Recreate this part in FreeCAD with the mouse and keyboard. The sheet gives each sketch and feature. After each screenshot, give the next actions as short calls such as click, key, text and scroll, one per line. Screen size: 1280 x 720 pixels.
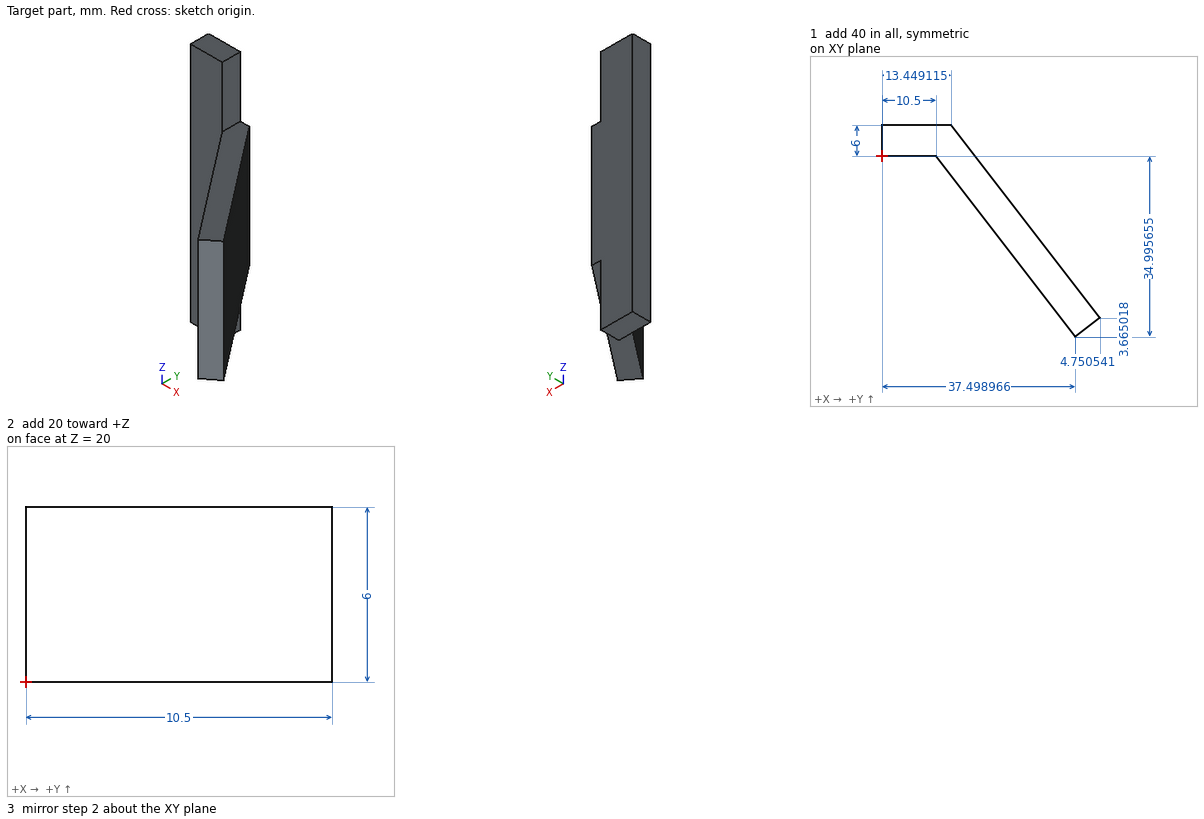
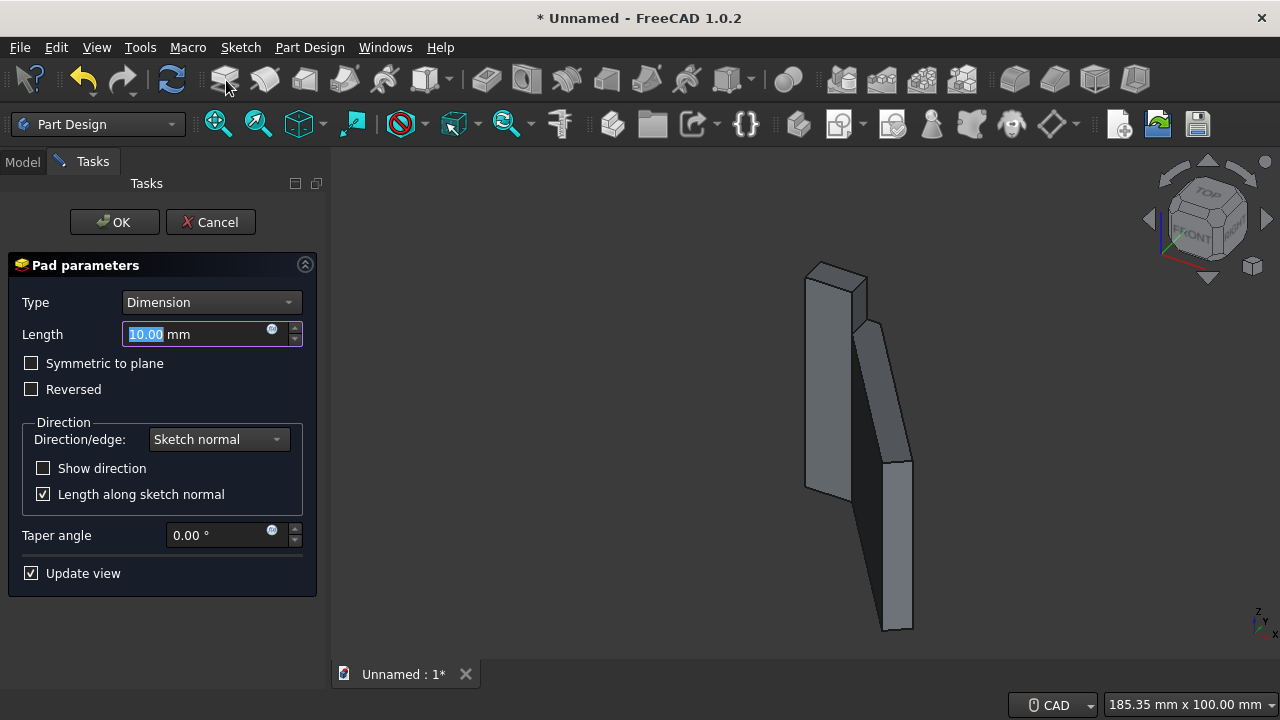
text(20)
key(Tab)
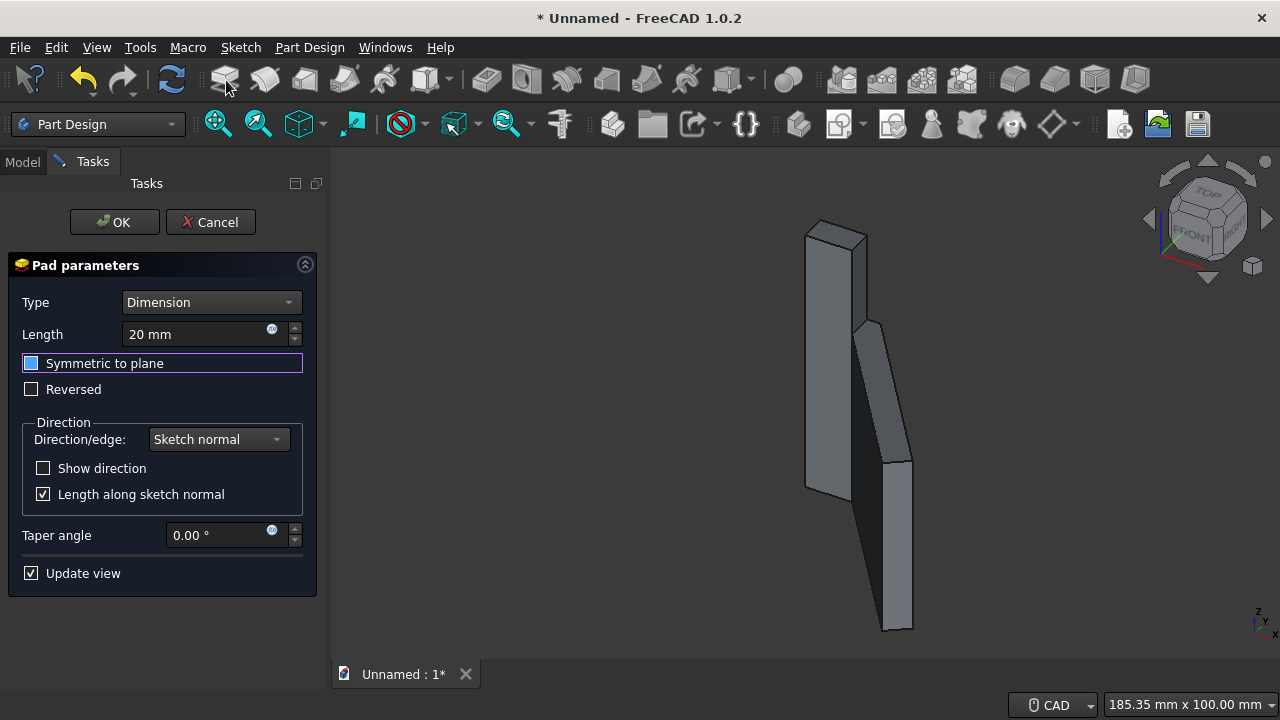
click(115, 222)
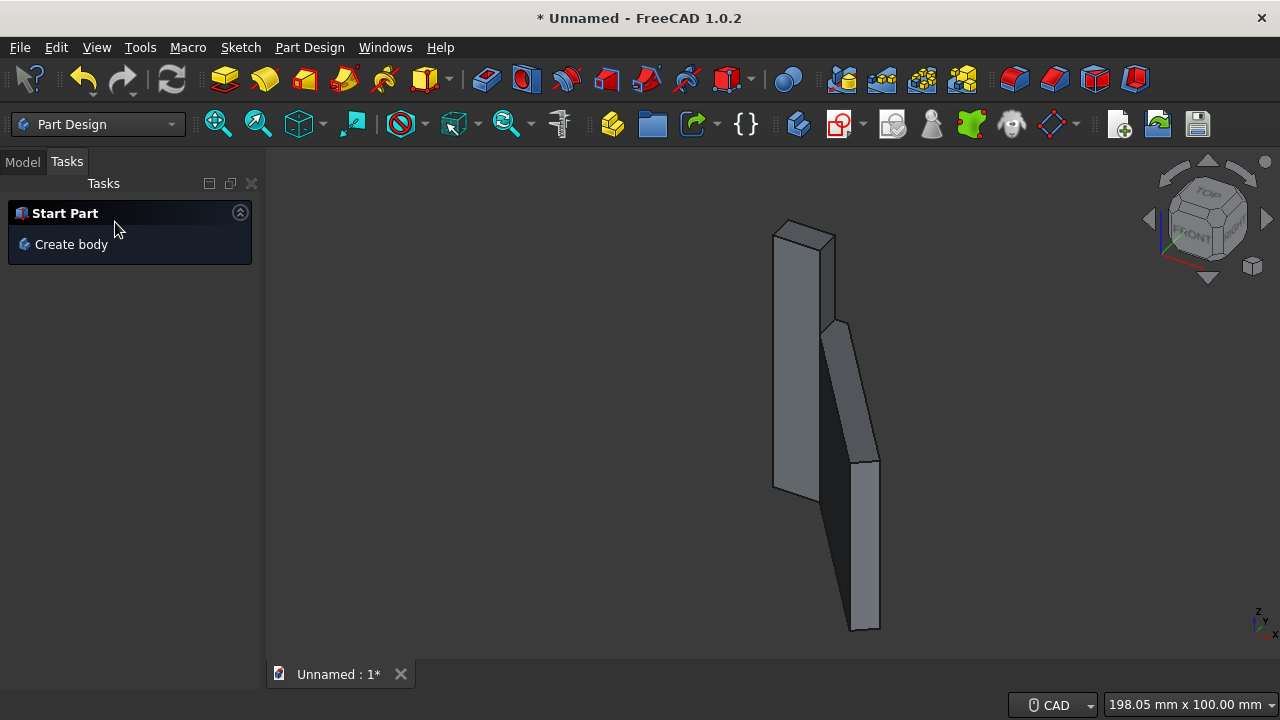
click(23, 161)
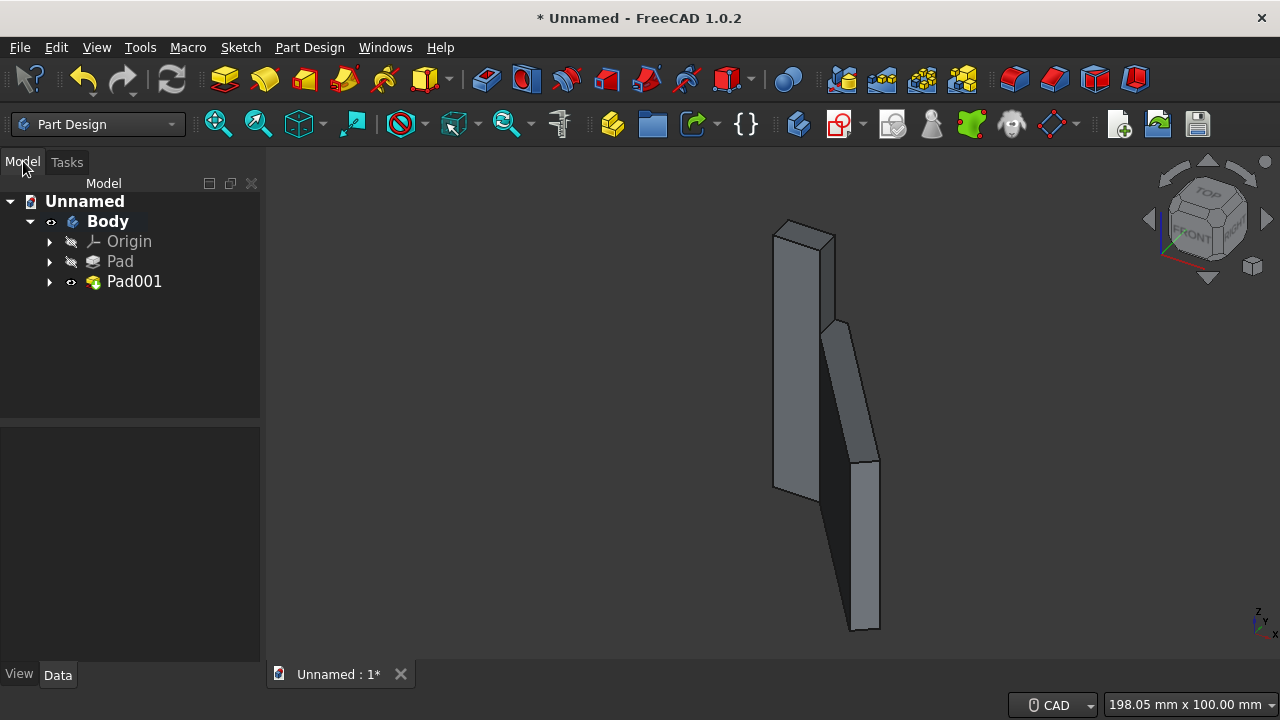
click(116, 282)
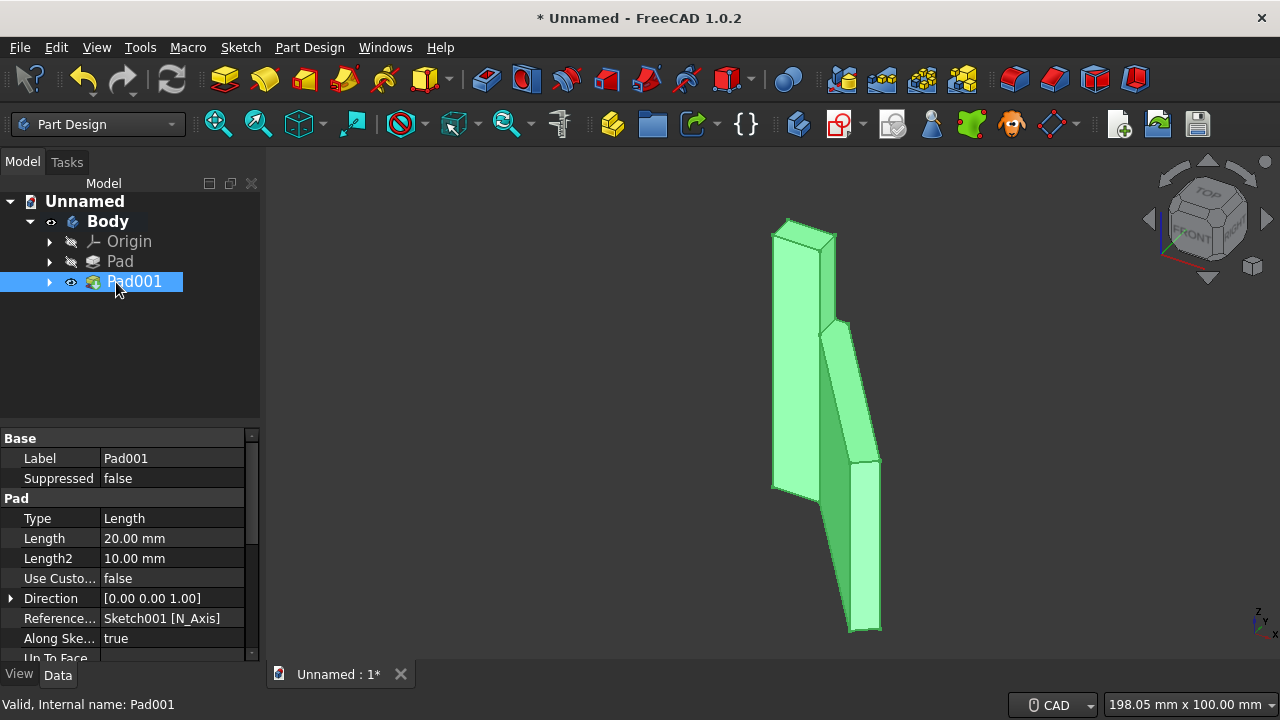
click(842, 80)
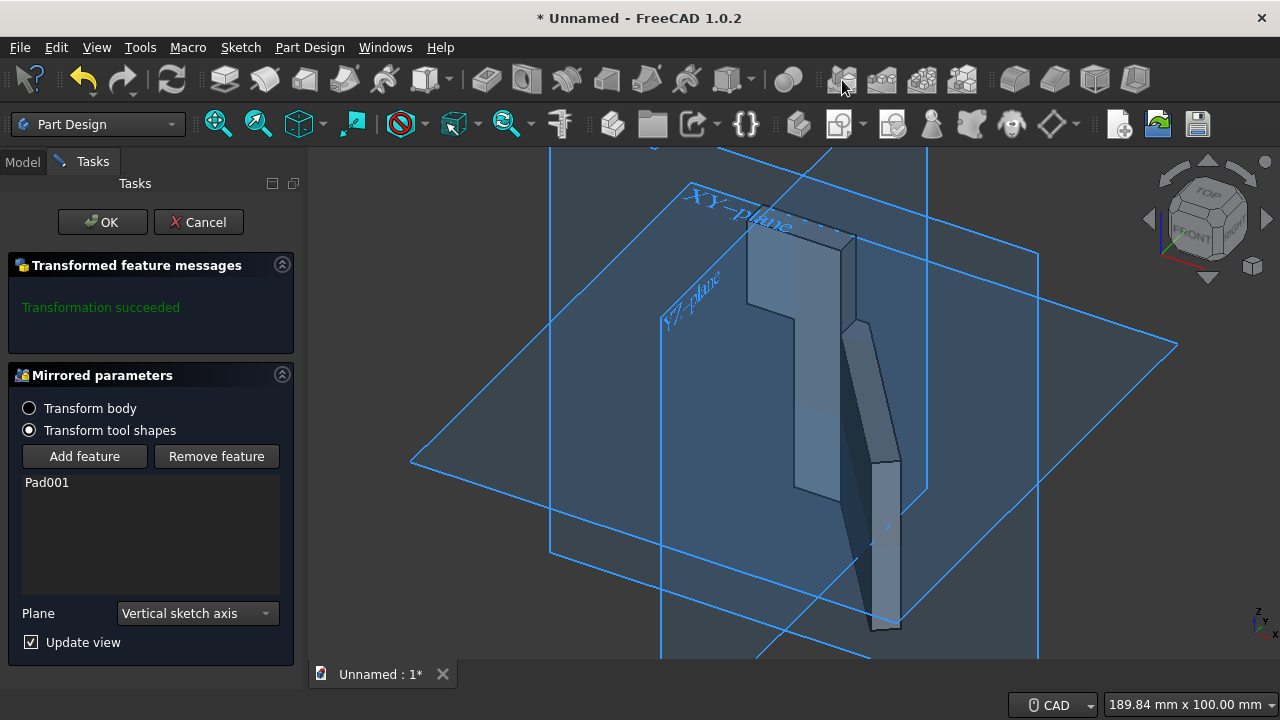
click(198, 614)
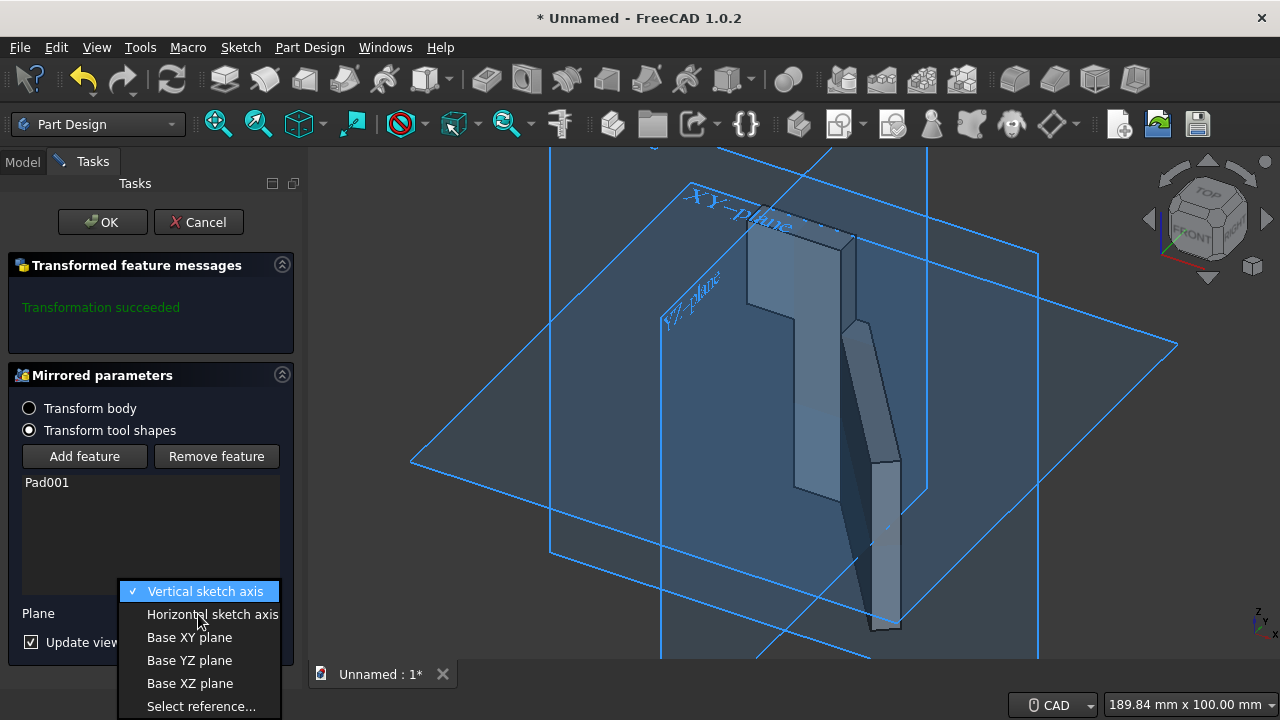
click(198, 638)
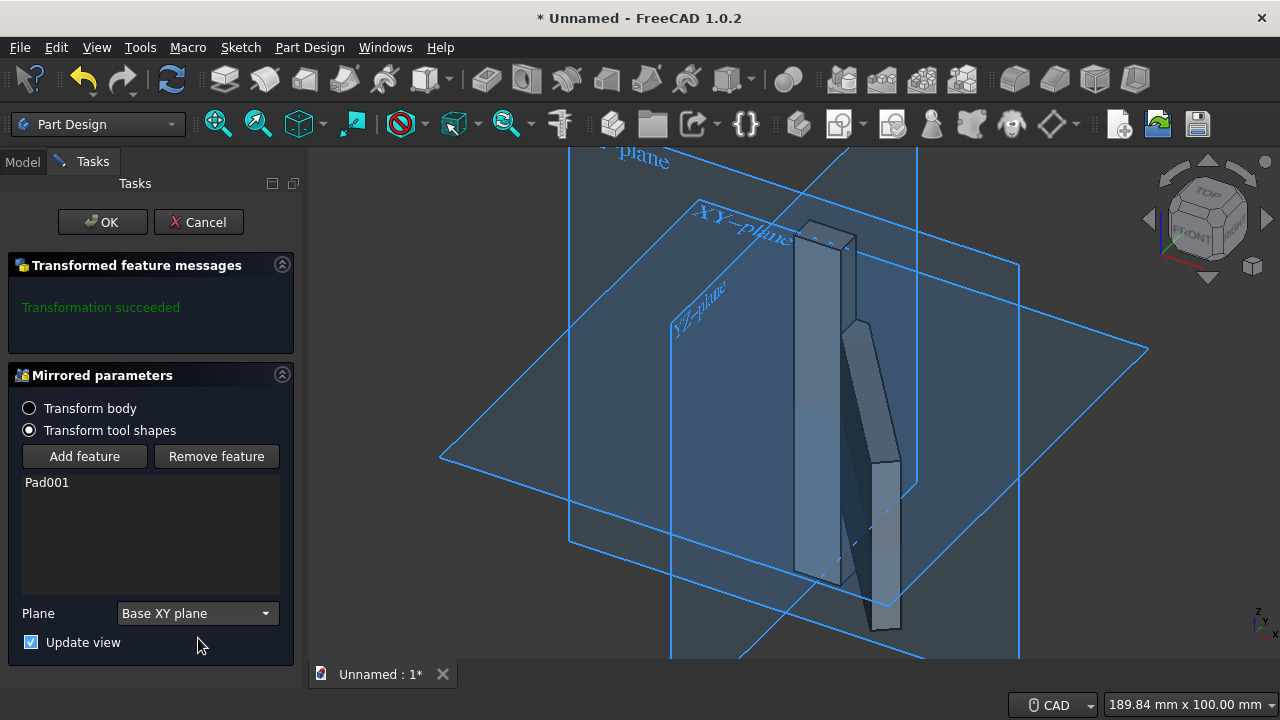
click(103, 222)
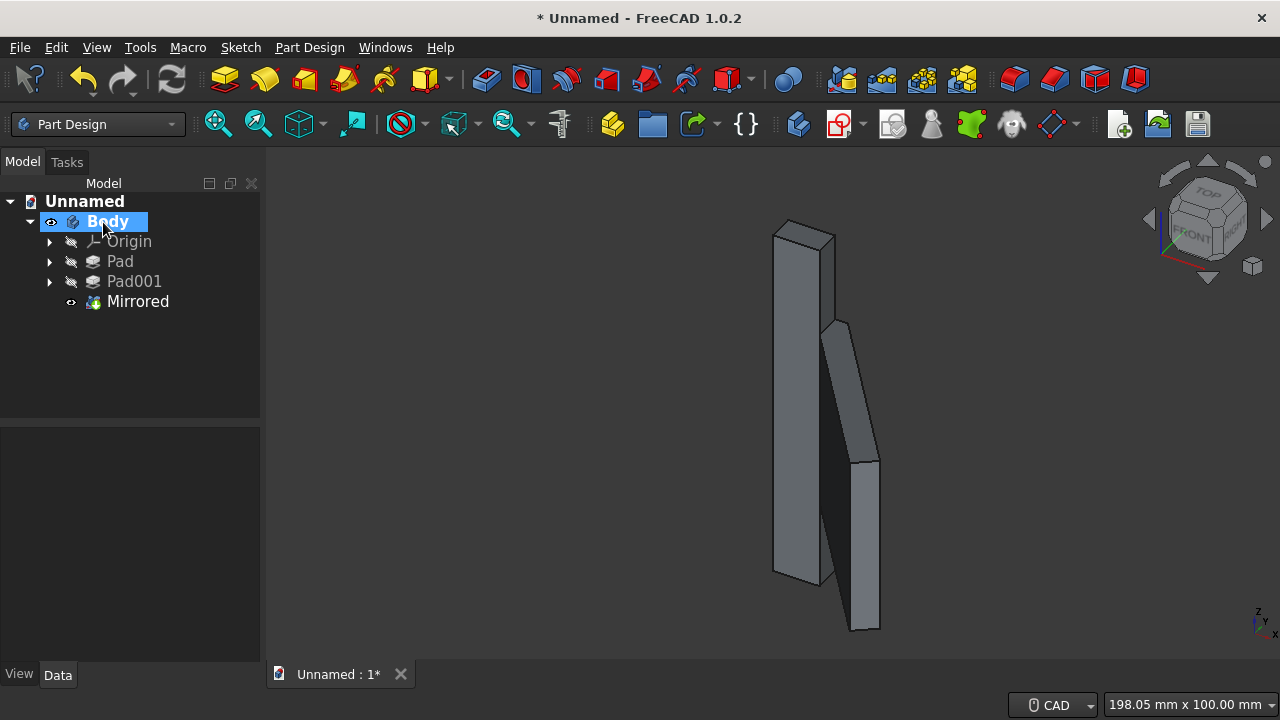
key(0)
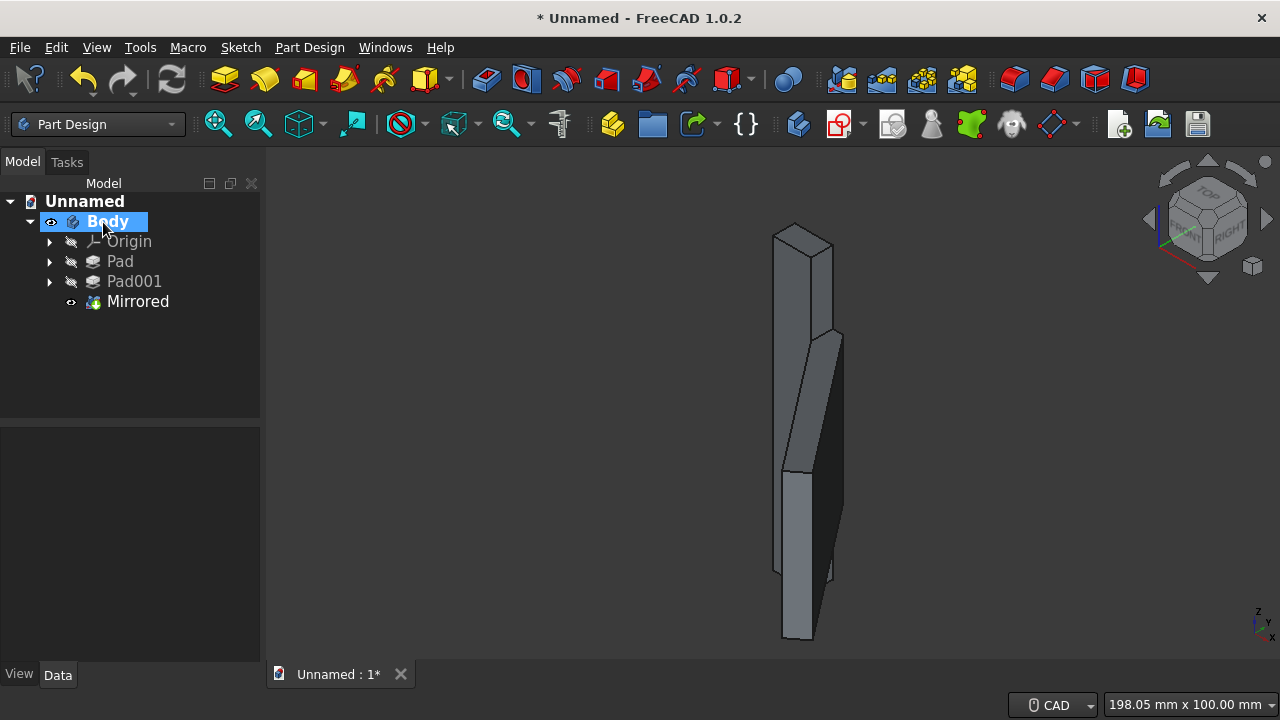
click(220, 124)